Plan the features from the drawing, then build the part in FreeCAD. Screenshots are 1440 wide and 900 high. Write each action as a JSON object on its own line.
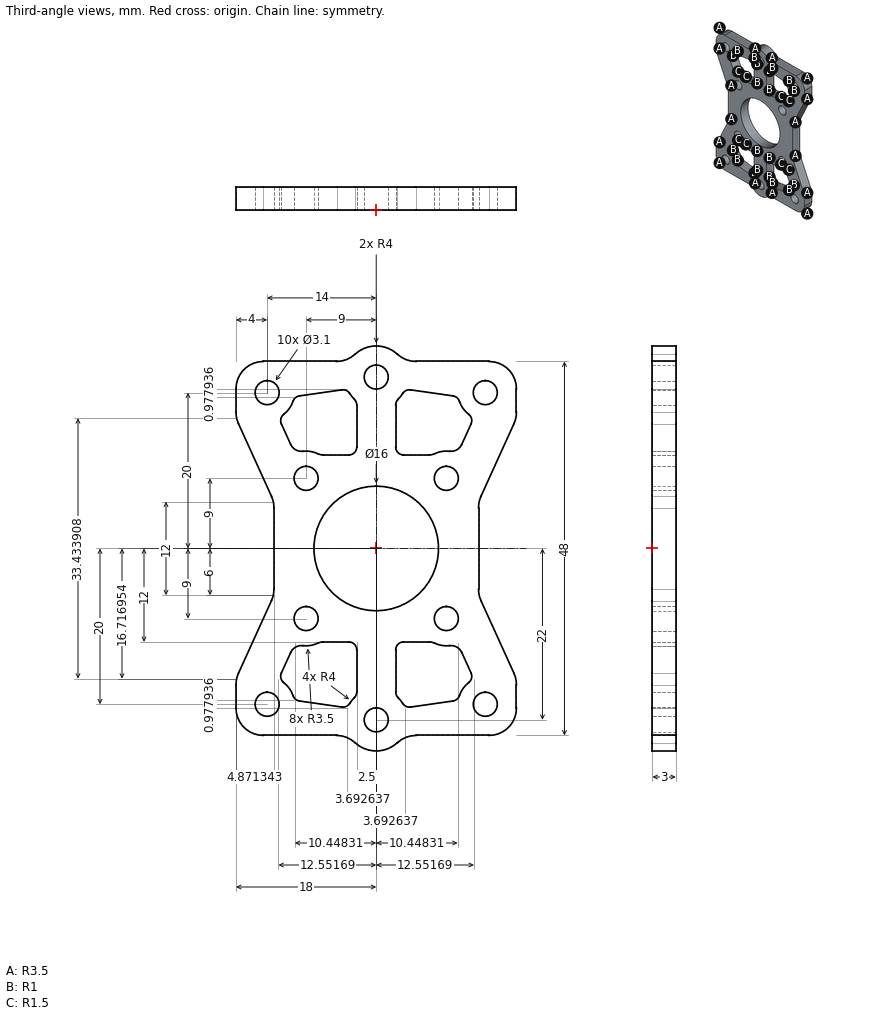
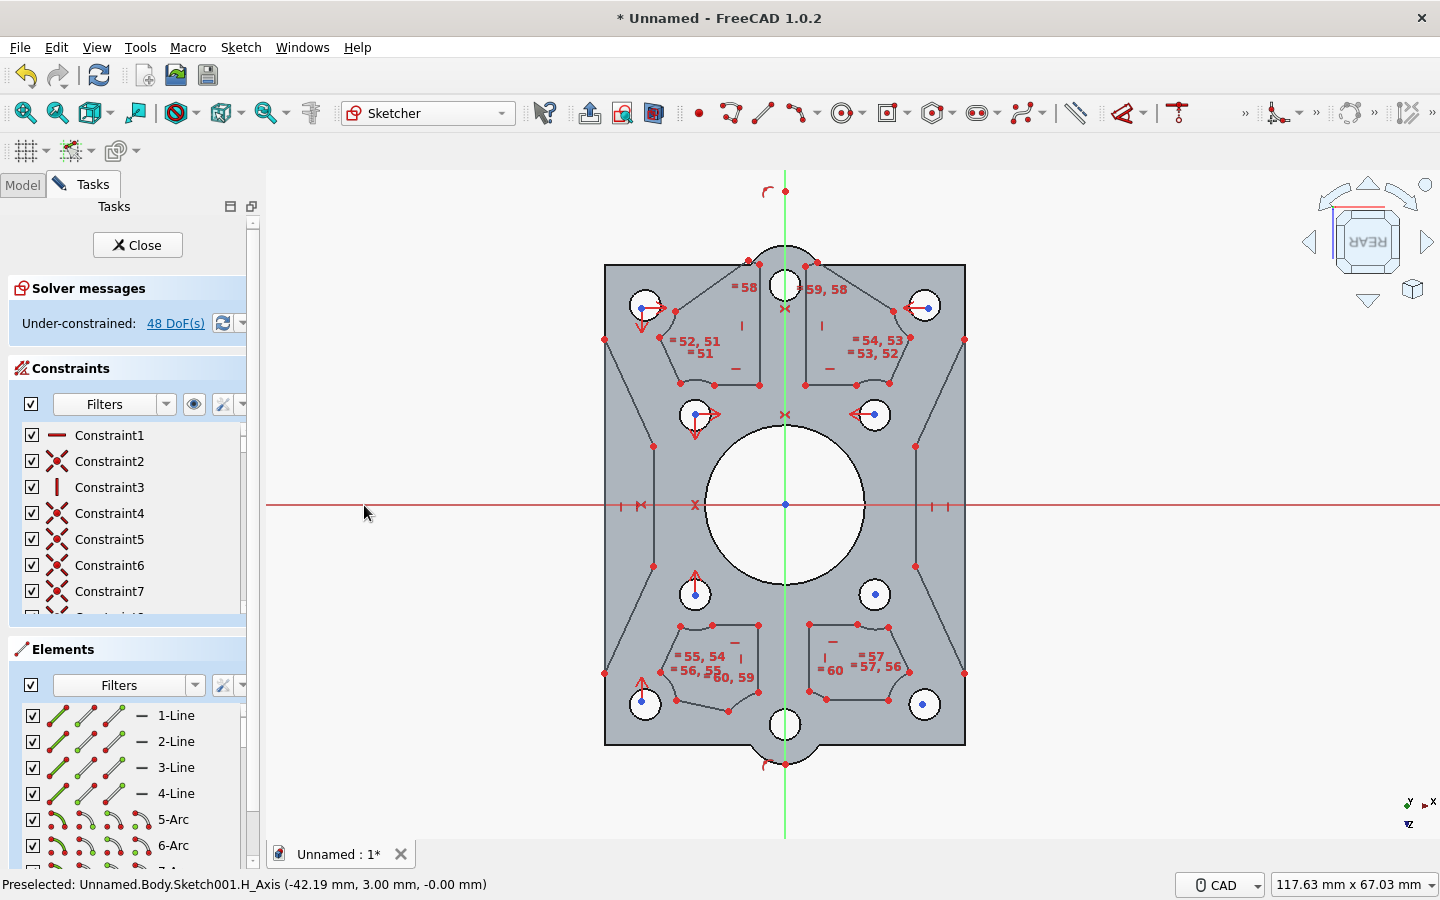
{"action": "left_click", "coordinate": [928, 308]}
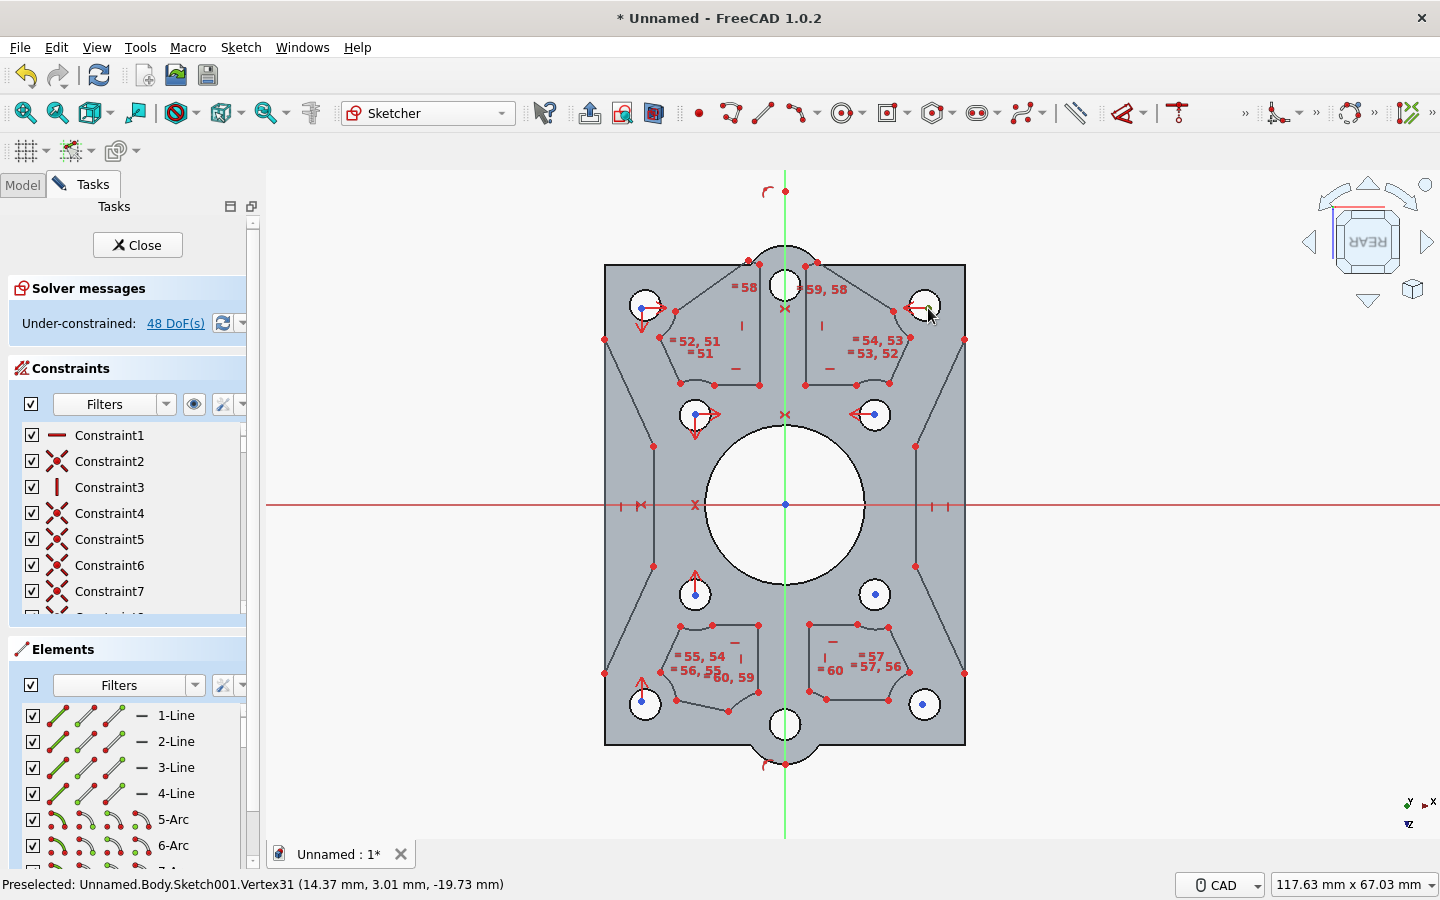
{"action": "left_click", "coordinate": [923, 705]}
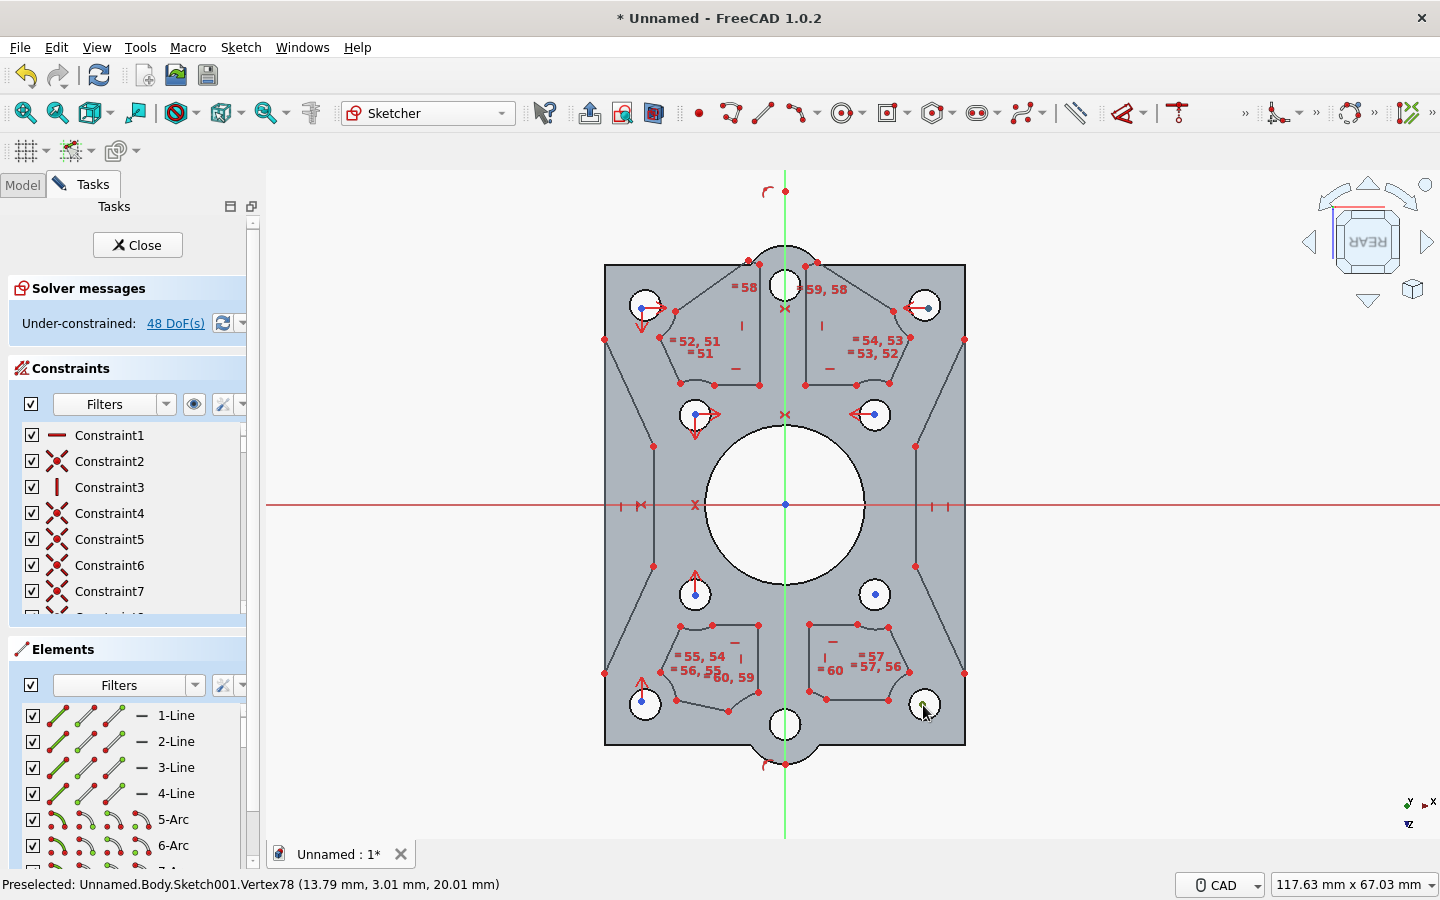
{"action": "left_click", "coordinate": [364, 505]}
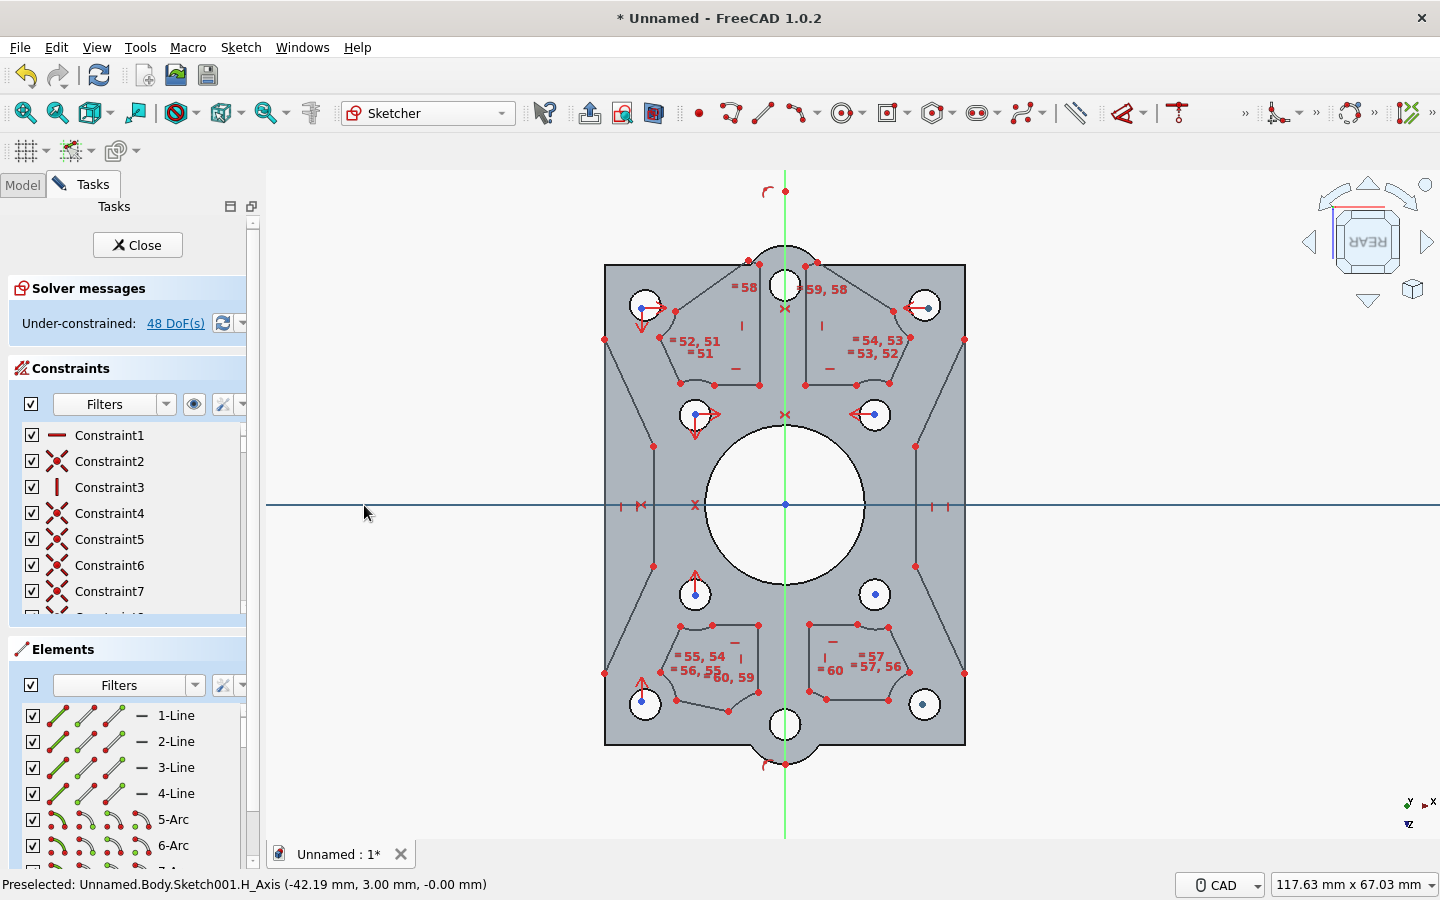
{"action": "key", "text": "s"}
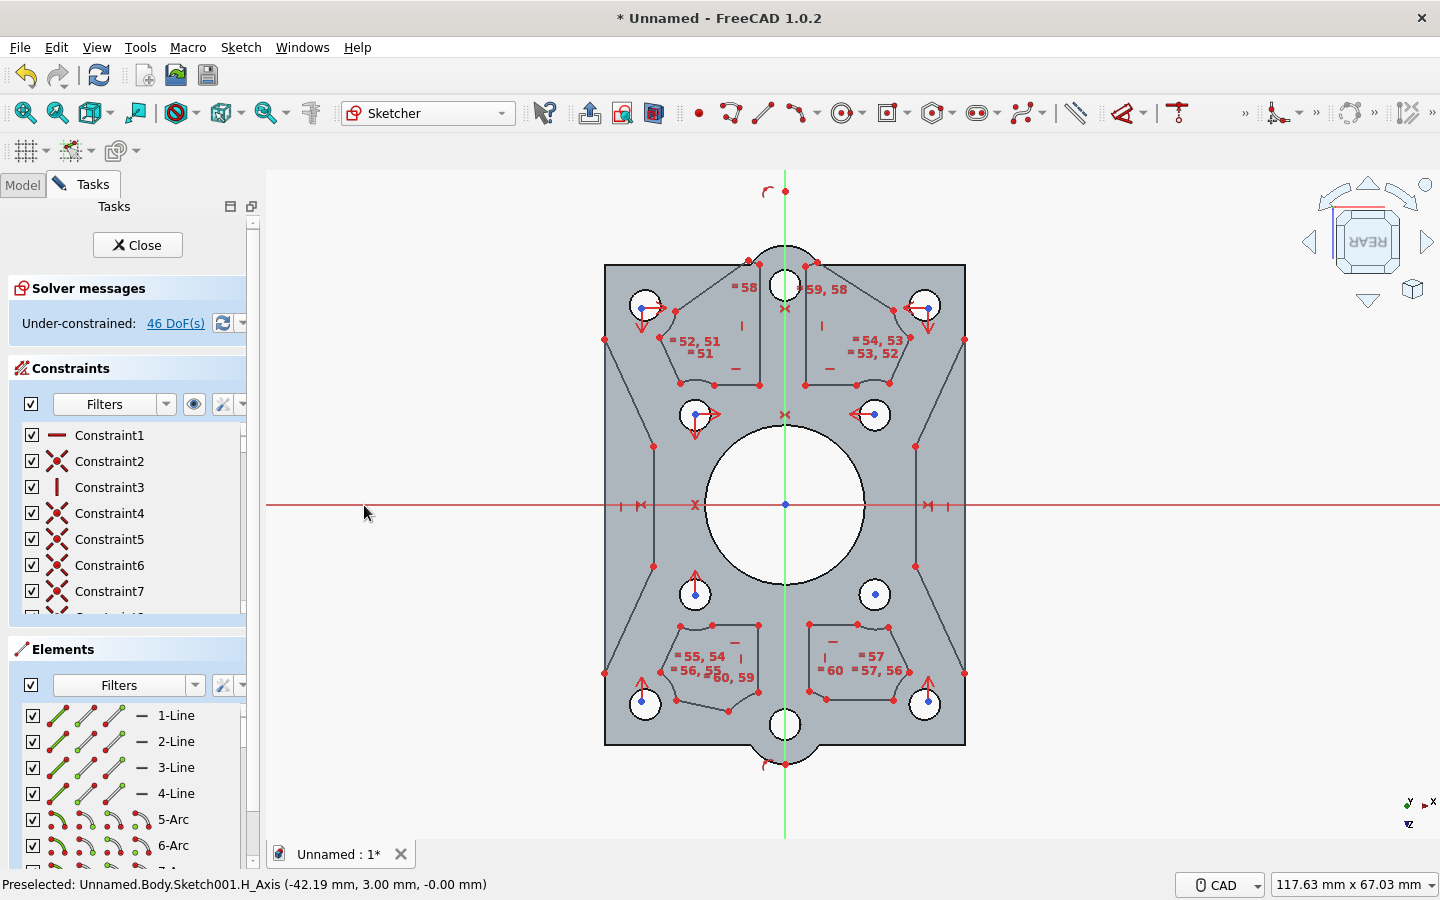
{"action": "left_click", "coordinate": [875, 414]}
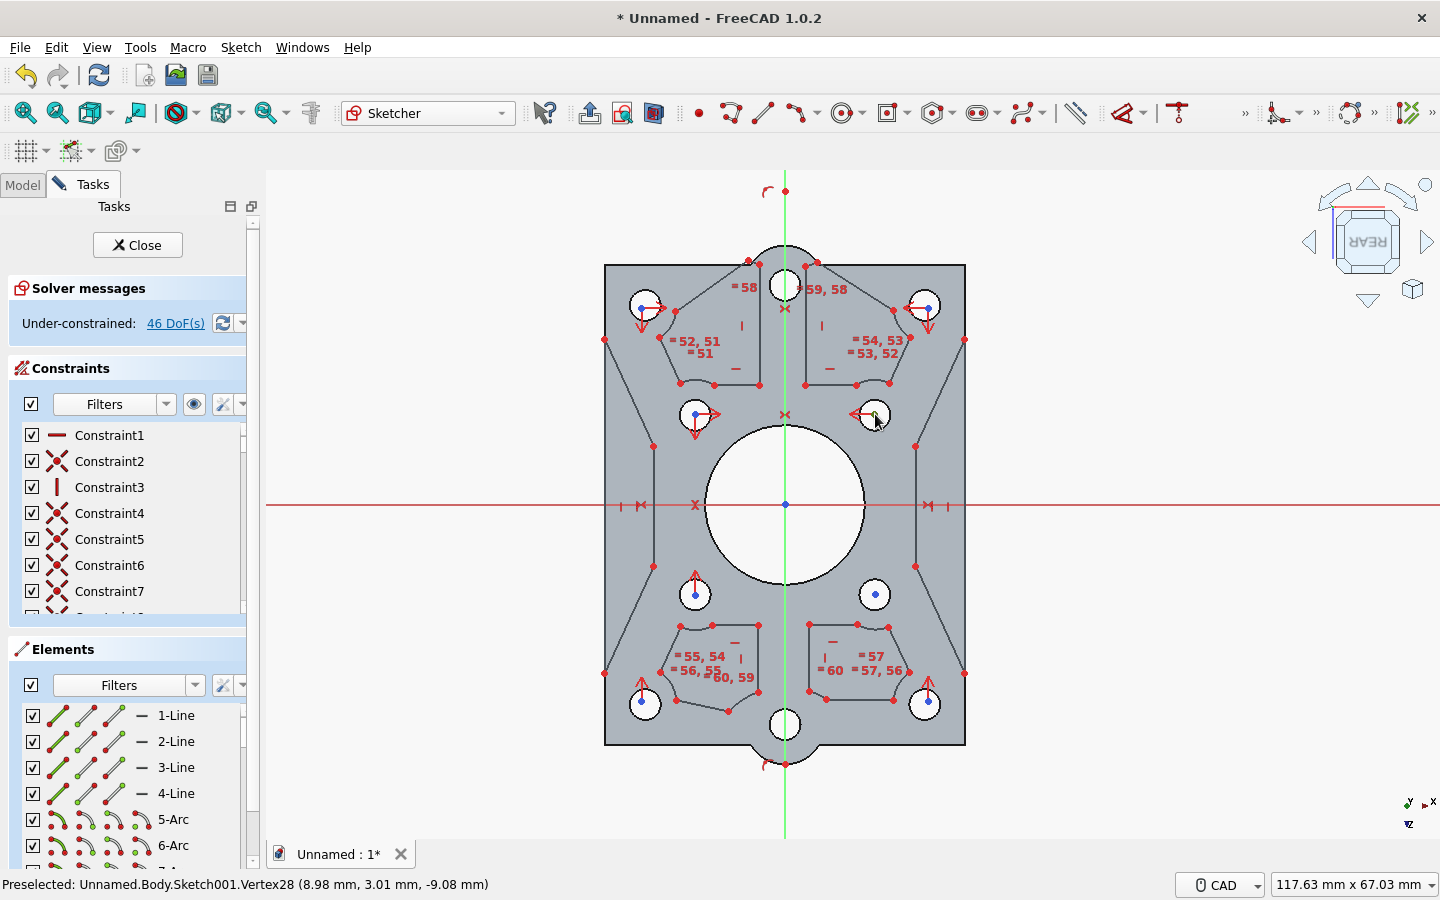
{"action": "left_click", "coordinate": [876, 595]}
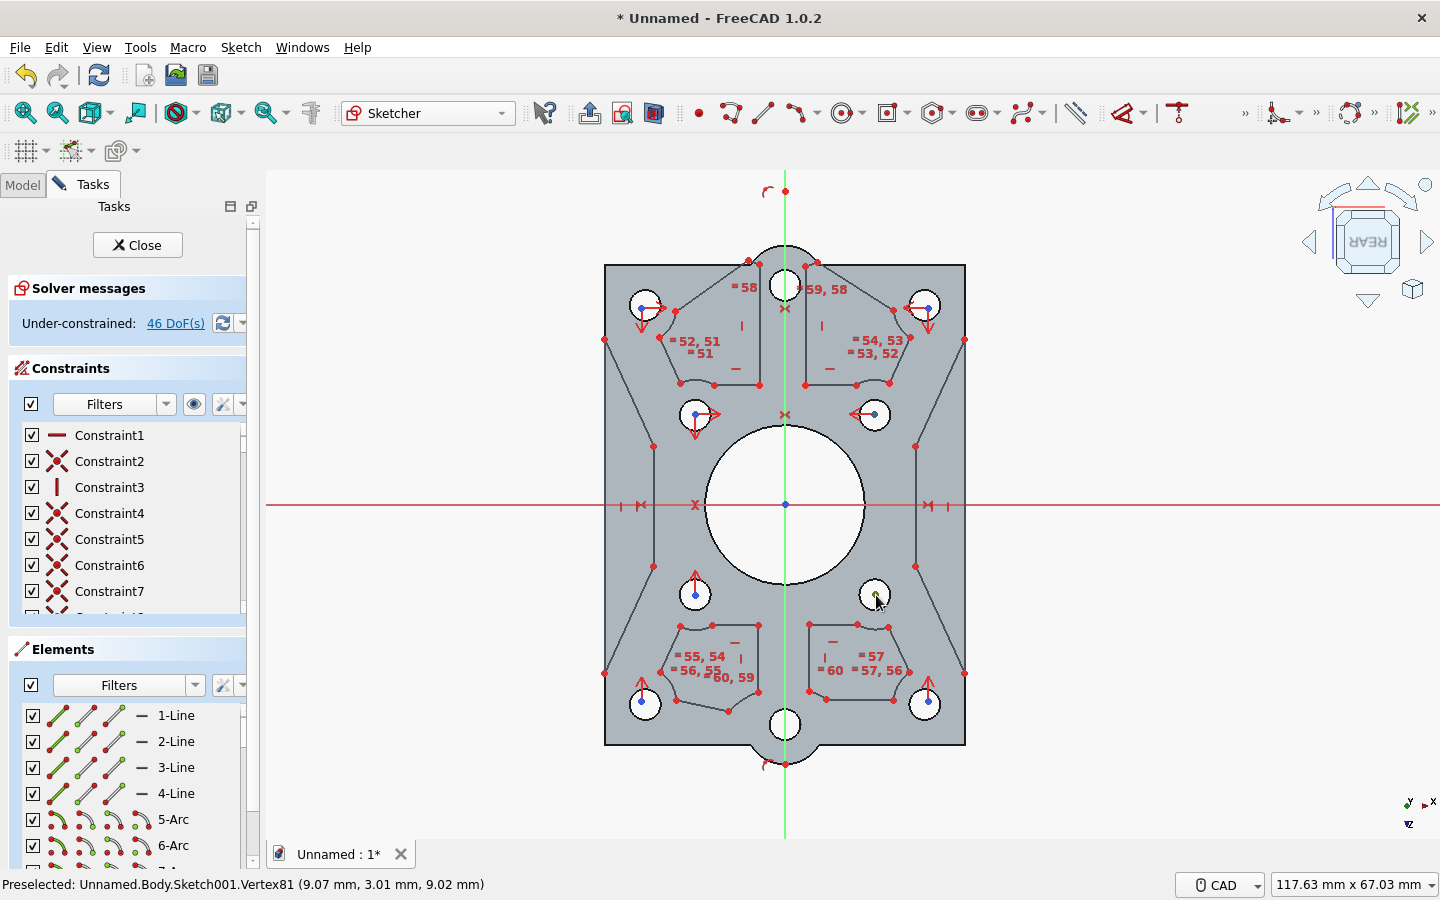
{"action": "left_click", "coordinate": [364, 505]}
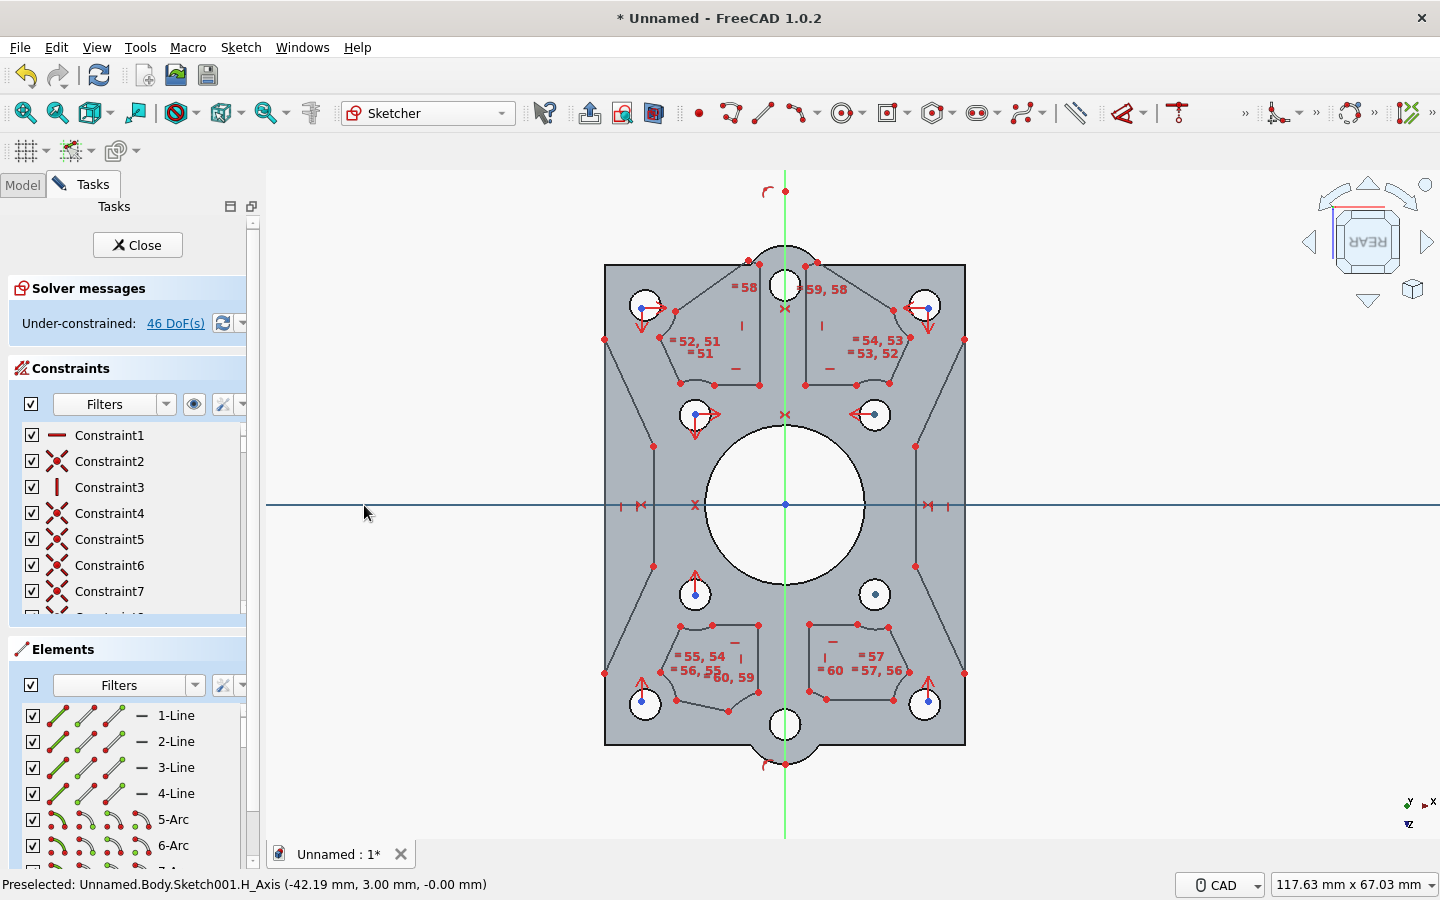
{"action": "key", "text": "s"}